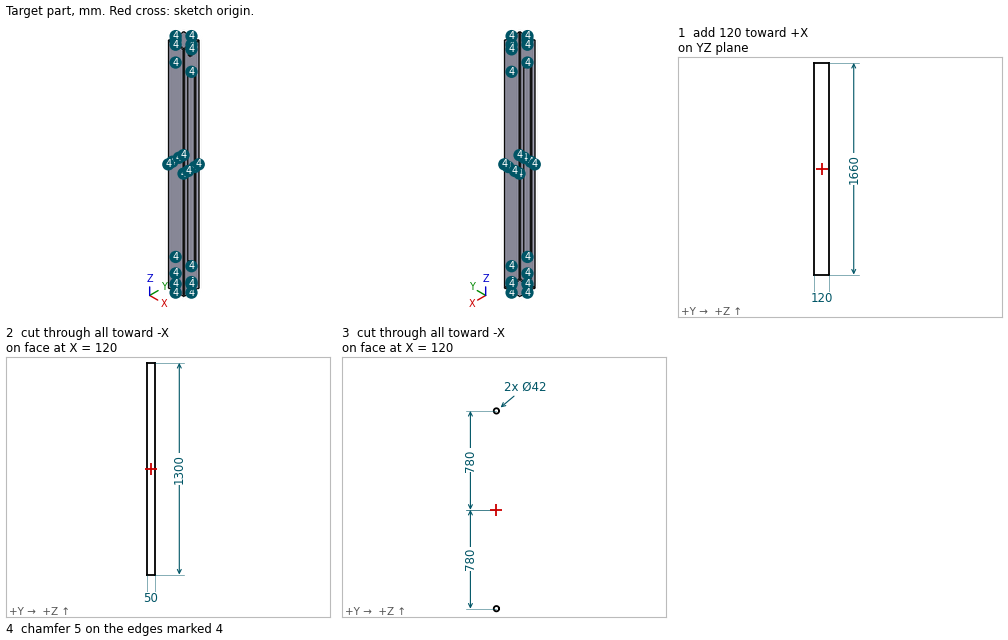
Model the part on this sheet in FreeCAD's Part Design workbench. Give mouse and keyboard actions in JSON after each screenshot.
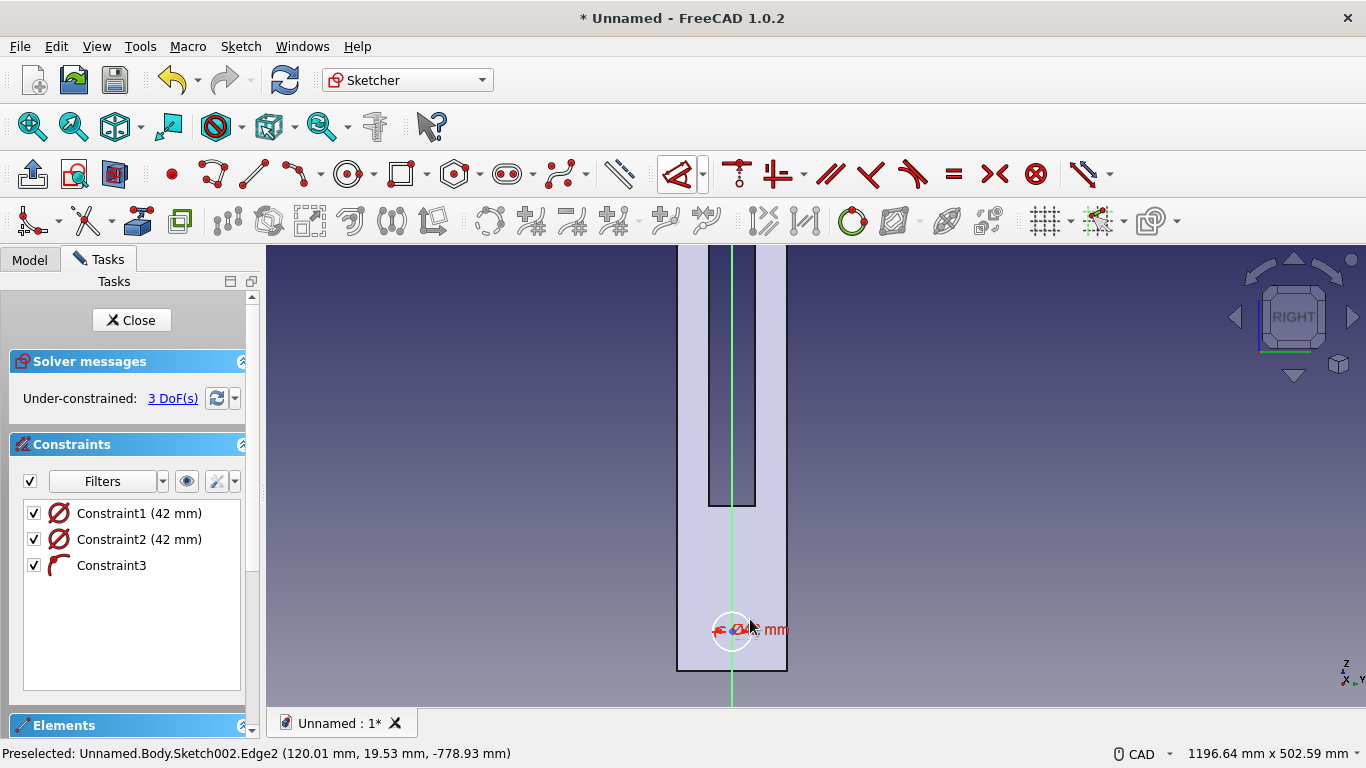
{"action": "scroll", "coordinate": [751, 620], "scroll_direction": "down", "scroll_amount": 8}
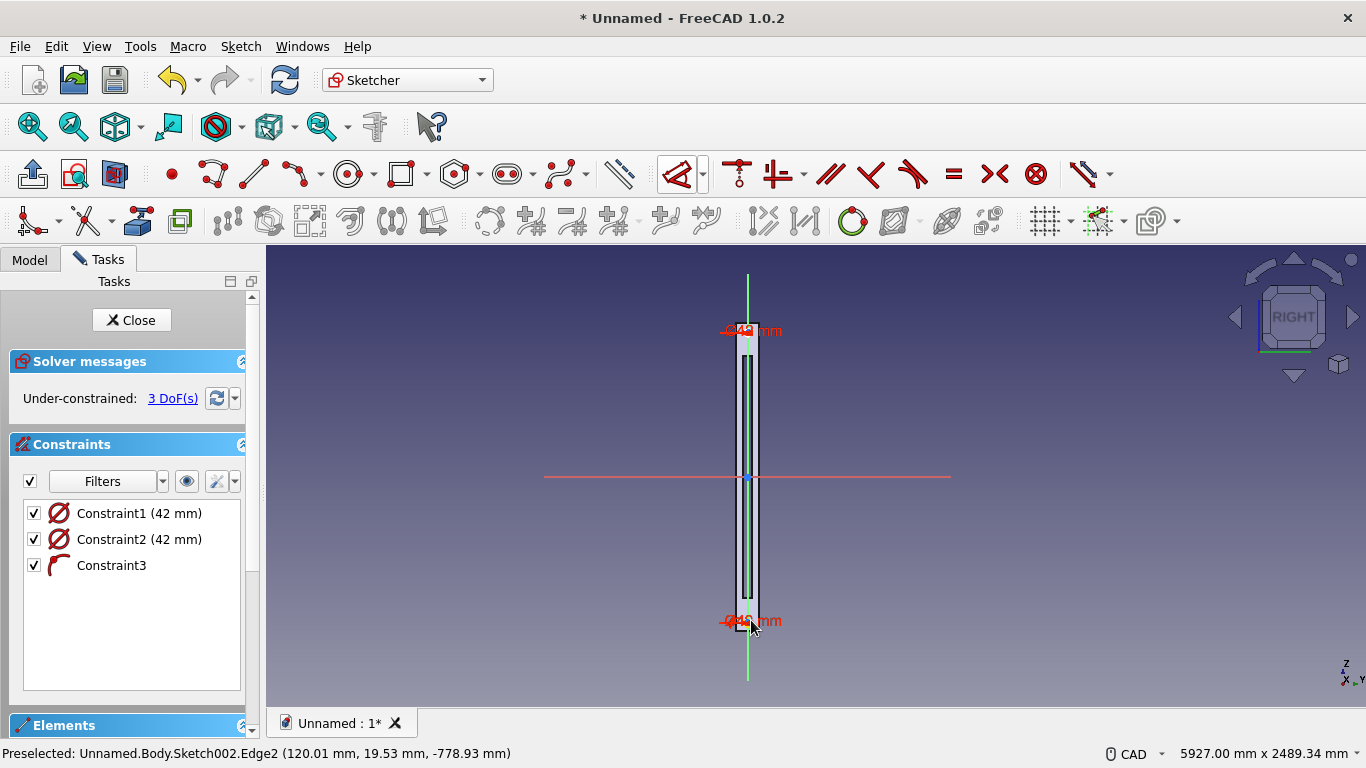
{"action": "left_click", "coordinate": [748, 333]}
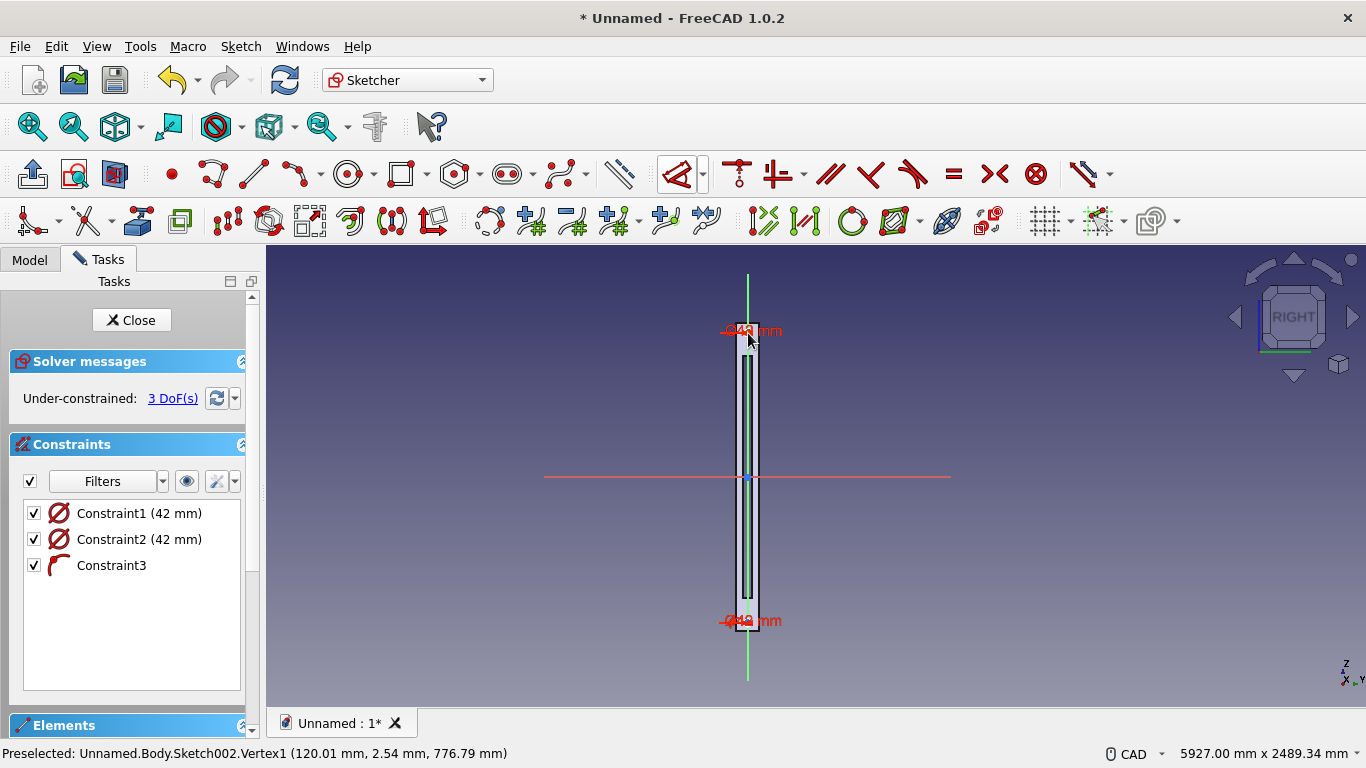
{"action": "left_click", "coordinate": [748, 563]}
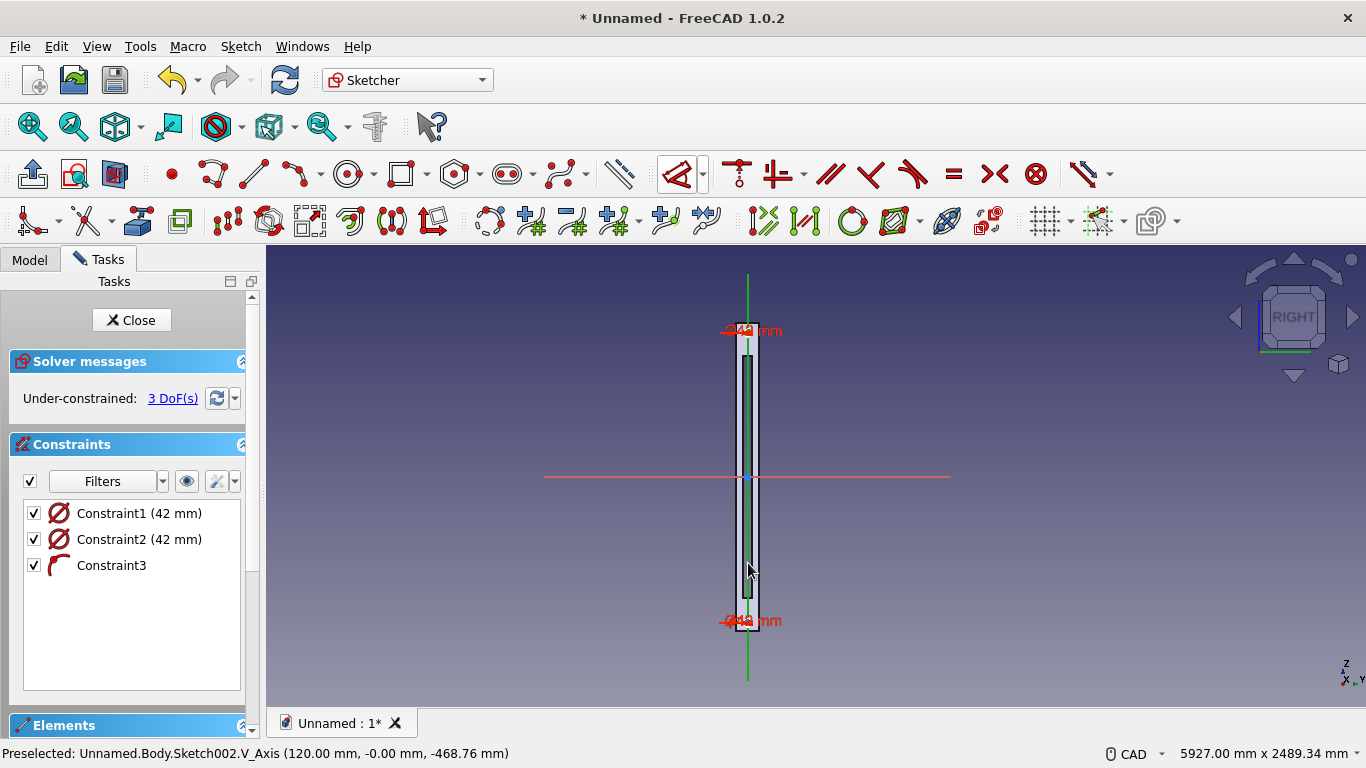
{"action": "key", "text": "c"}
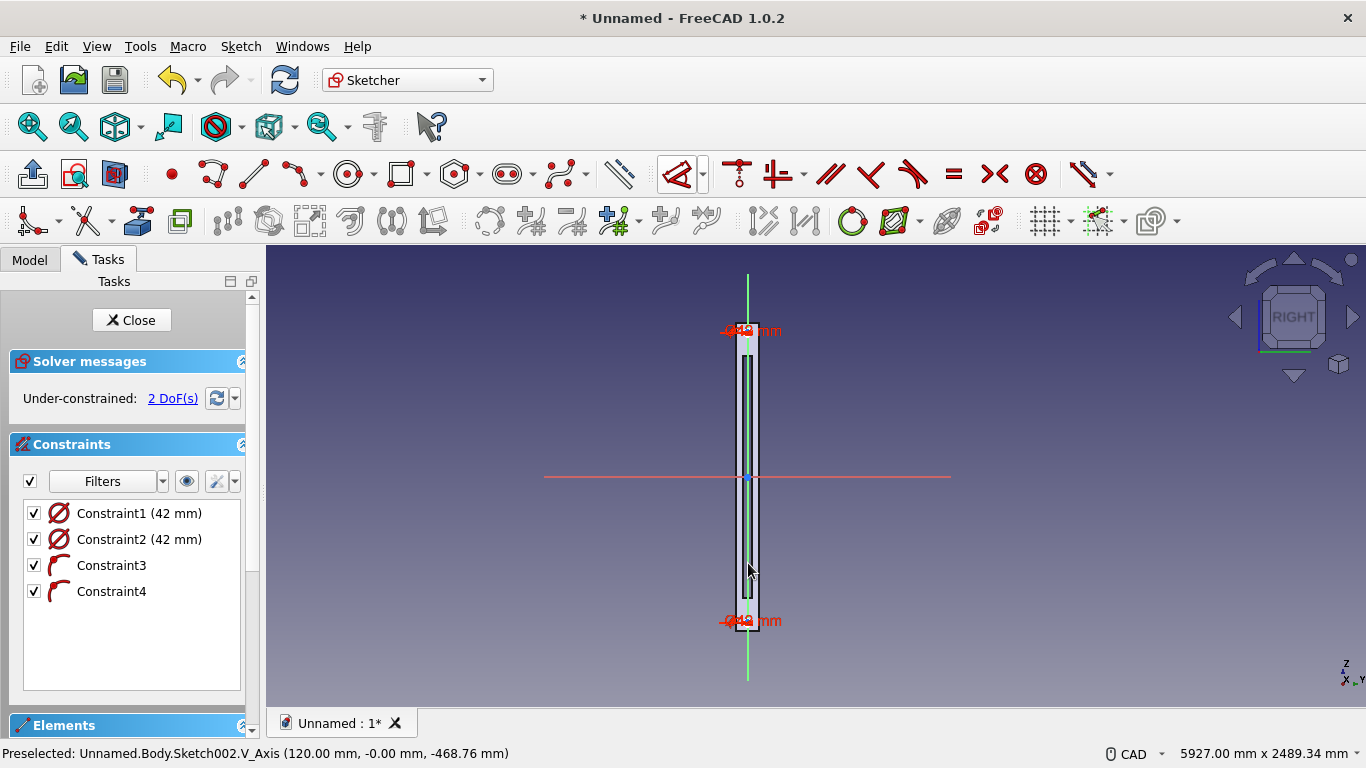
{"action": "left_click", "coordinate": [676, 174]}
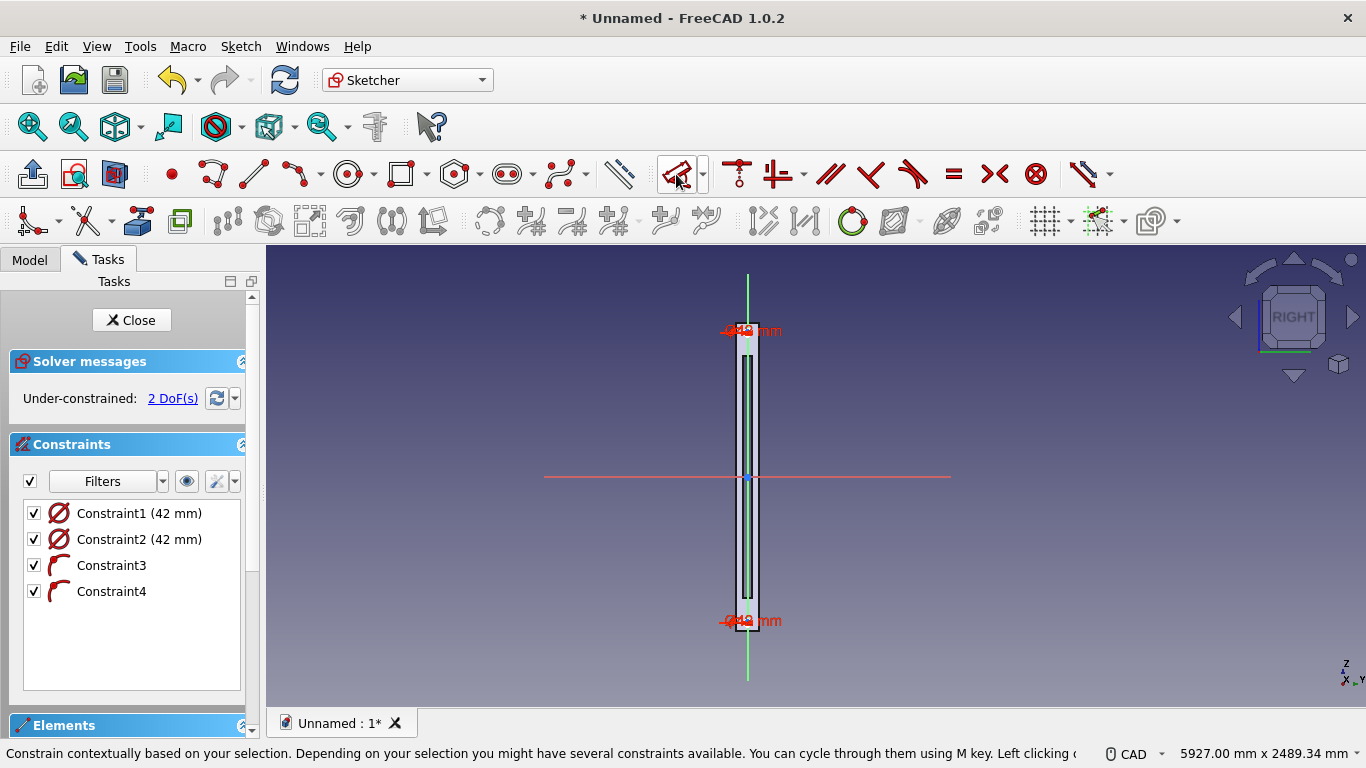
{"action": "left_click", "coordinate": [748, 333]}
{"action": "left_click", "coordinate": [782, 405]}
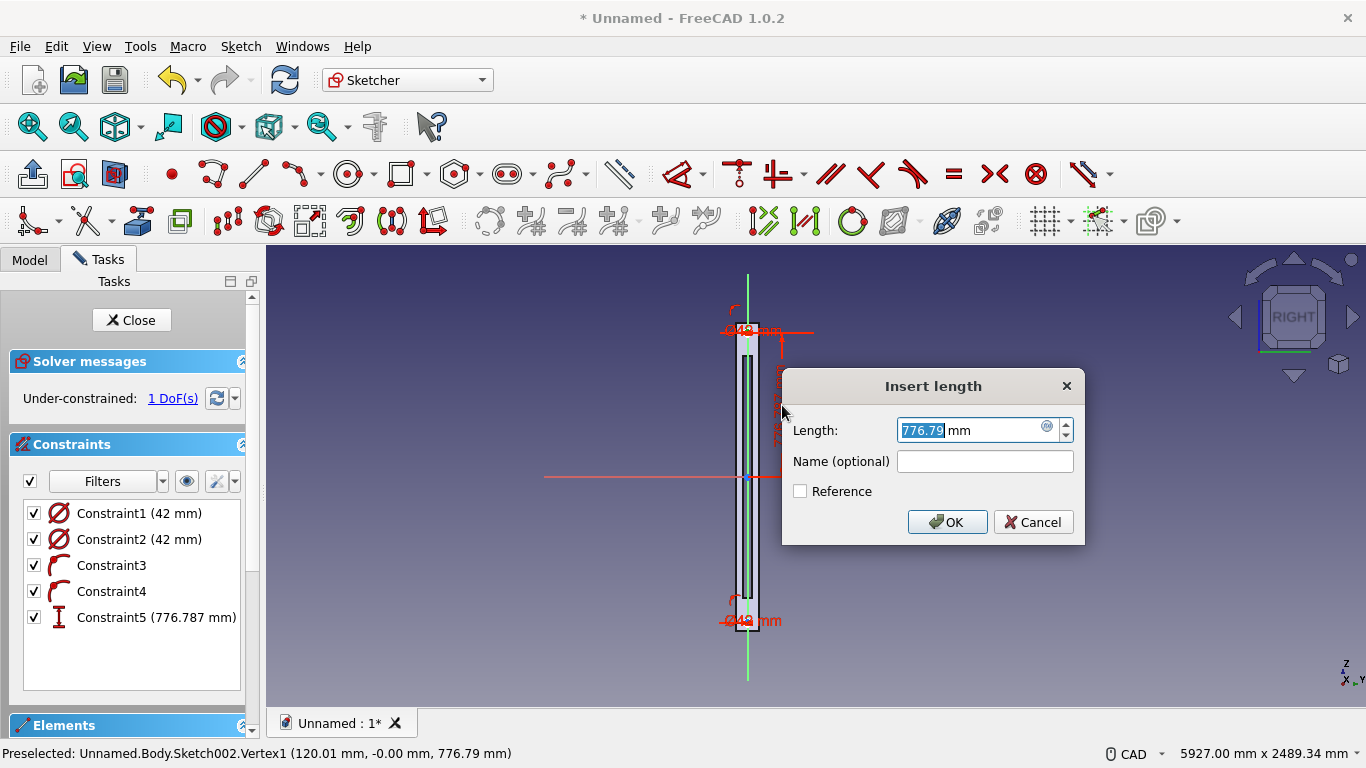
{"action": "type", "text": "780"}
{"action": "key", "text": "Return"}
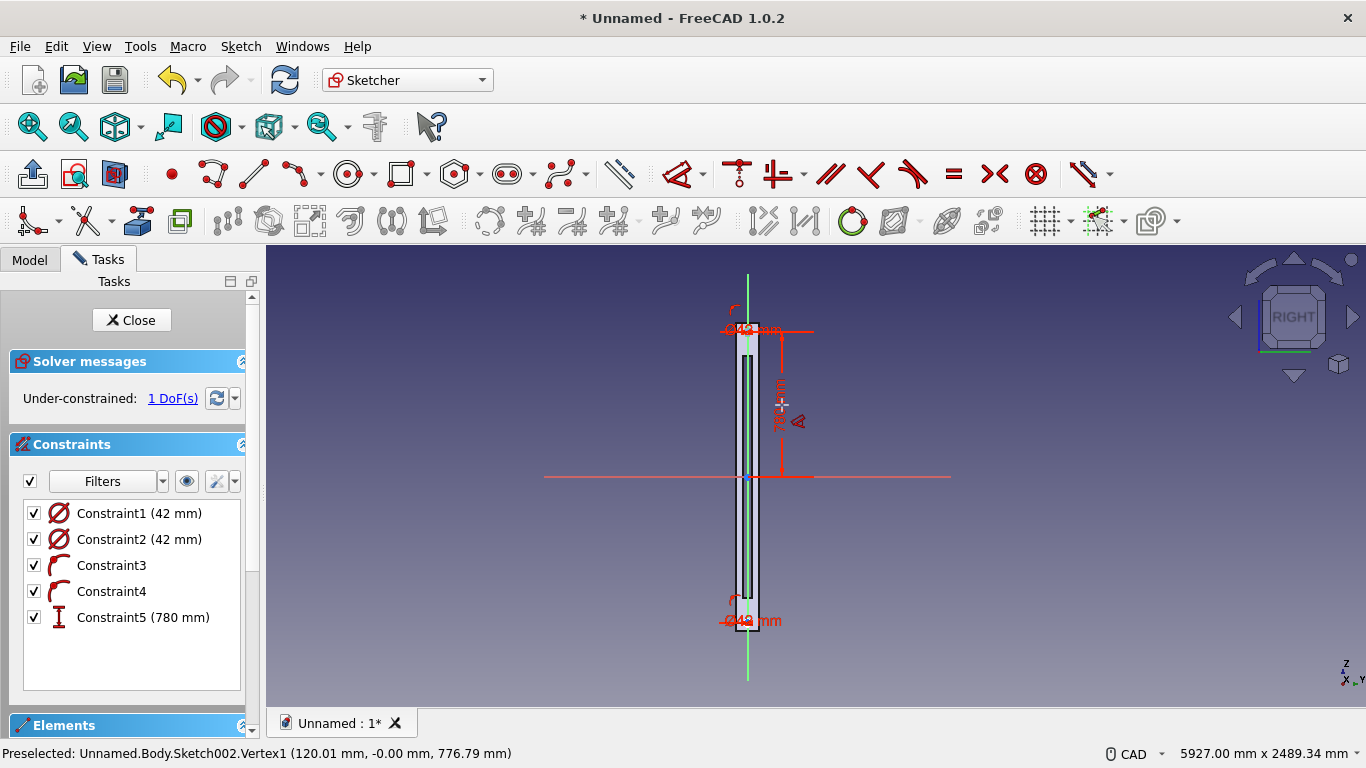
{"action": "left_click", "coordinate": [748, 623]}
{"action": "left_click", "coordinate": [782, 550]}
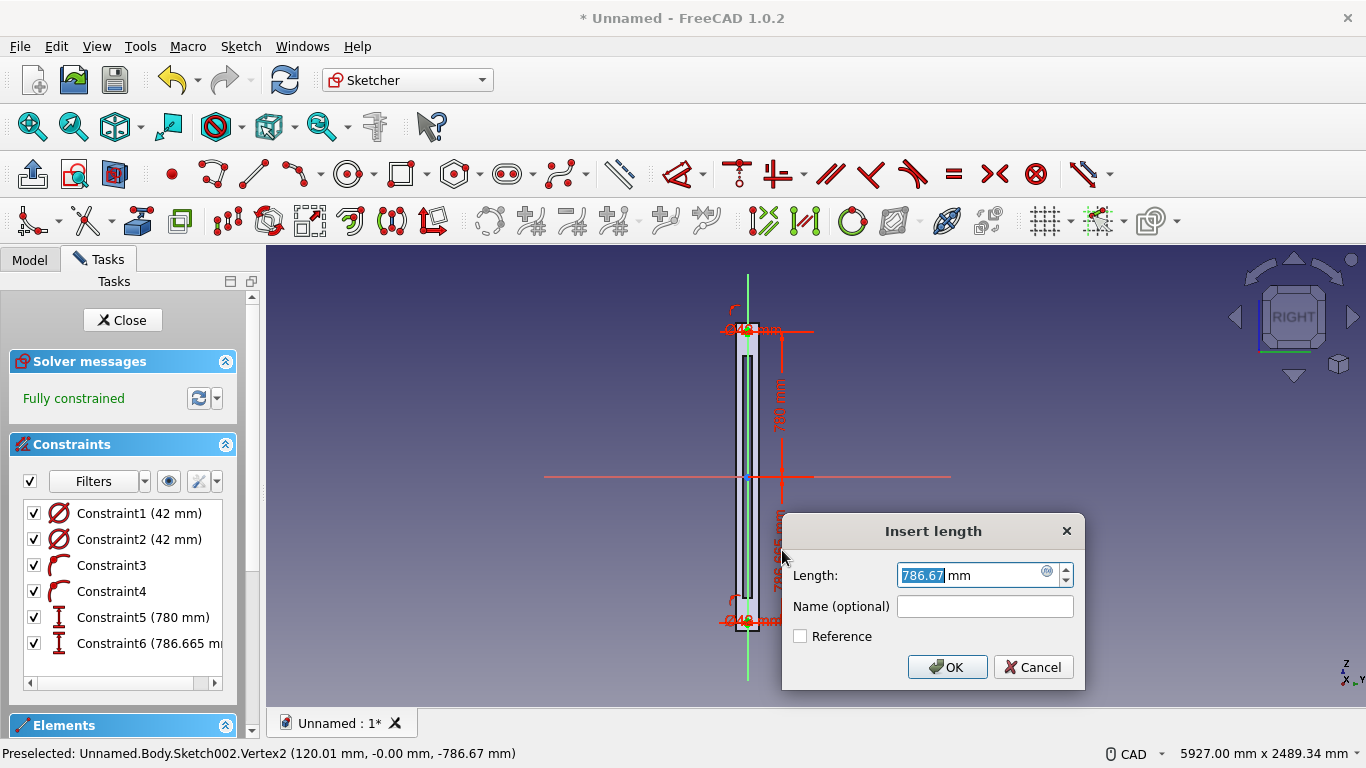
{"action": "type", "text": "780"}
{"action": "key", "text": "Return"}
{"action": "key", "text": "Escape"}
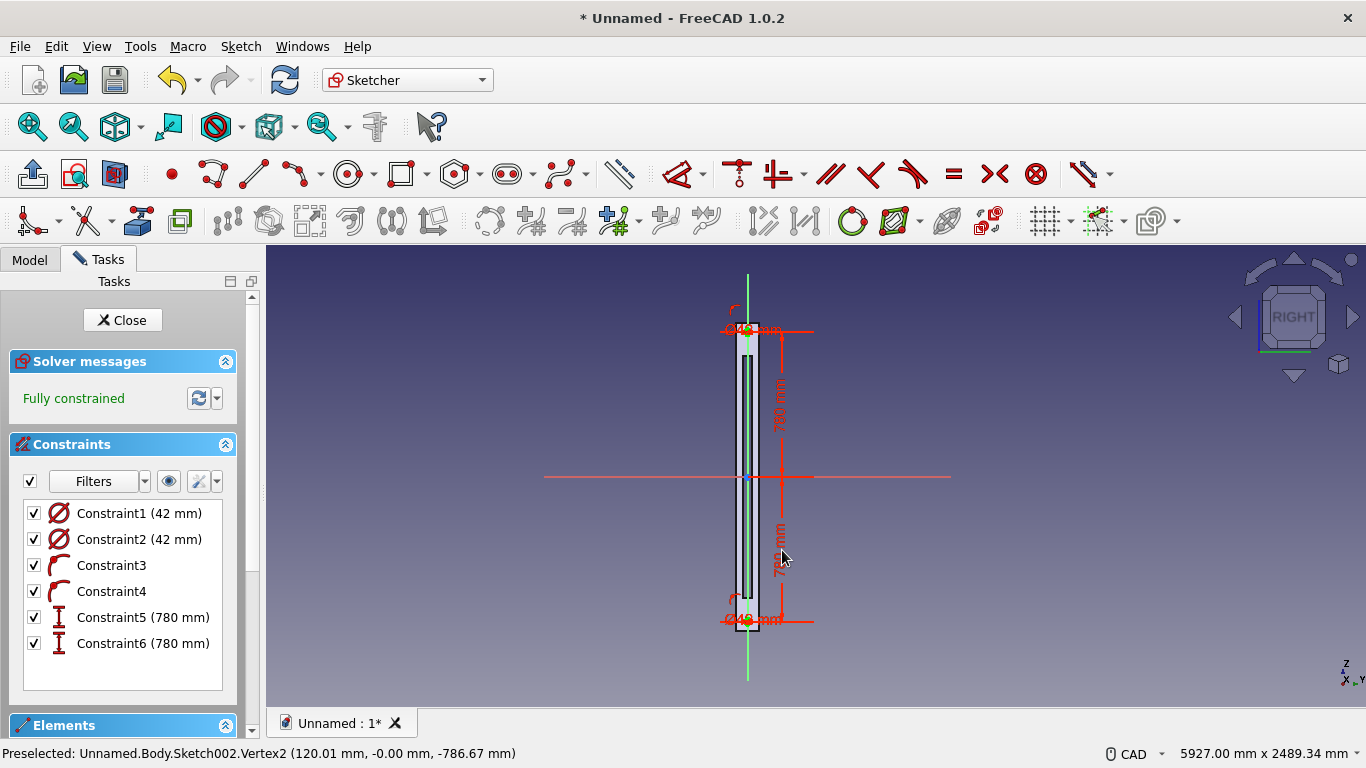
{"action": "left_click", "coordinate": [123, 320]}